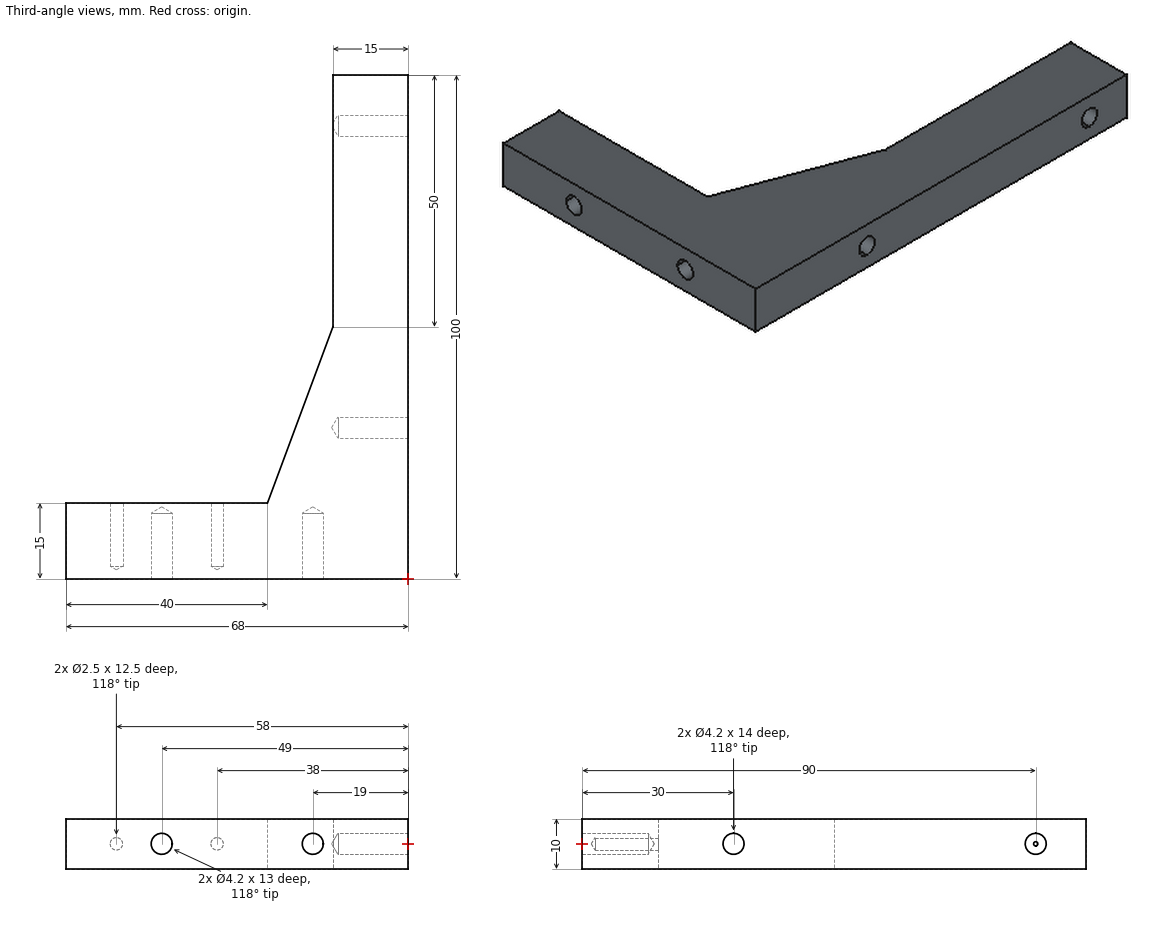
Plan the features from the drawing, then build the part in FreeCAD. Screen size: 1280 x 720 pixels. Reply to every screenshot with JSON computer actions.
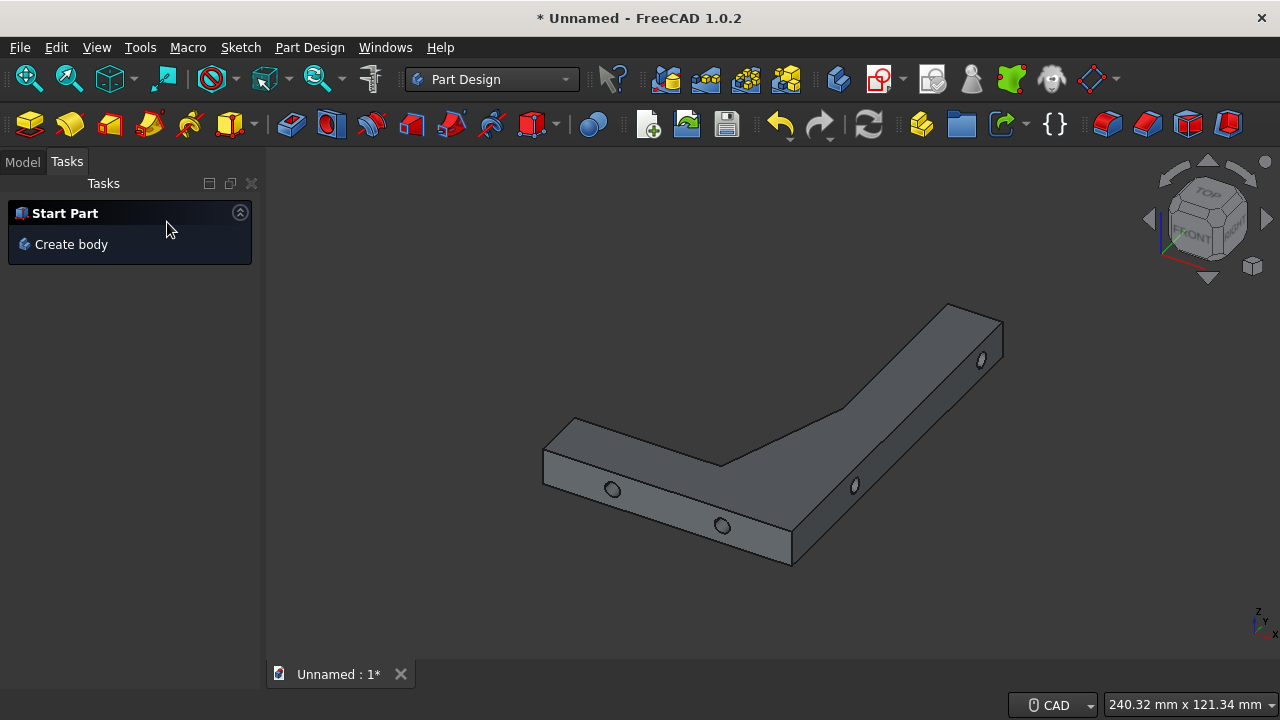
{"action": "key", "text": "4"}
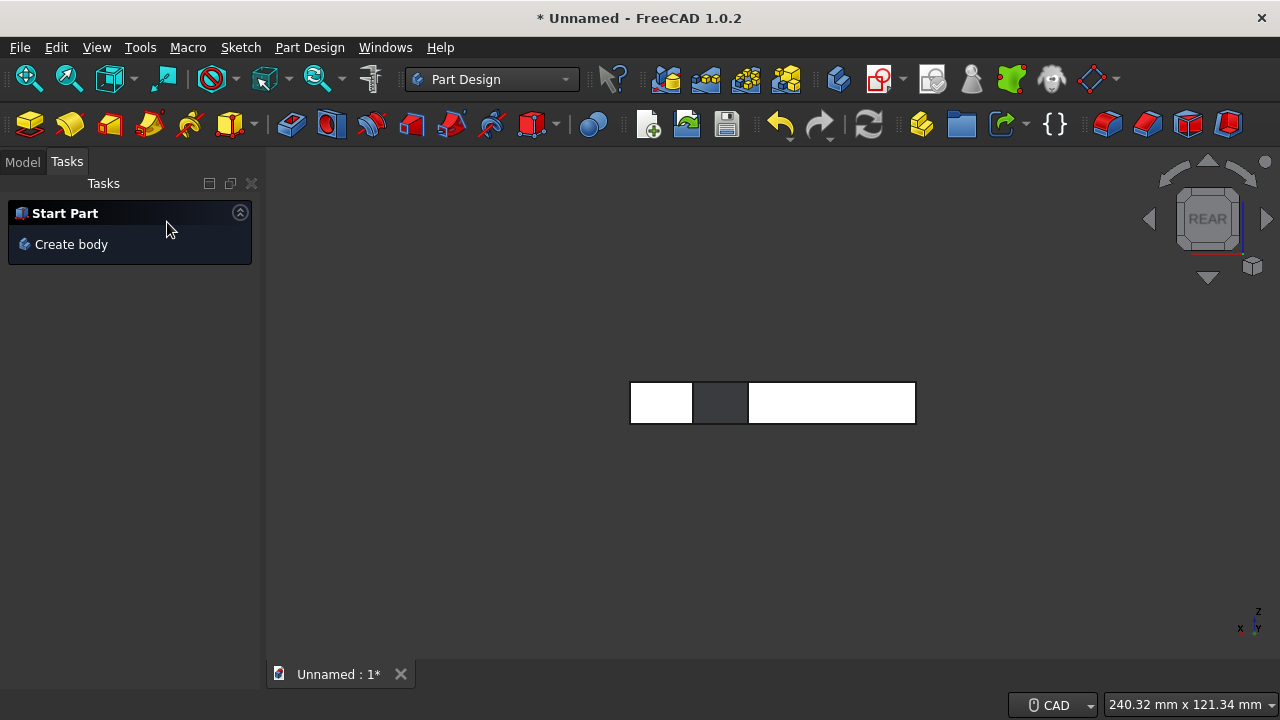
{"action": "key", "text": "v f"}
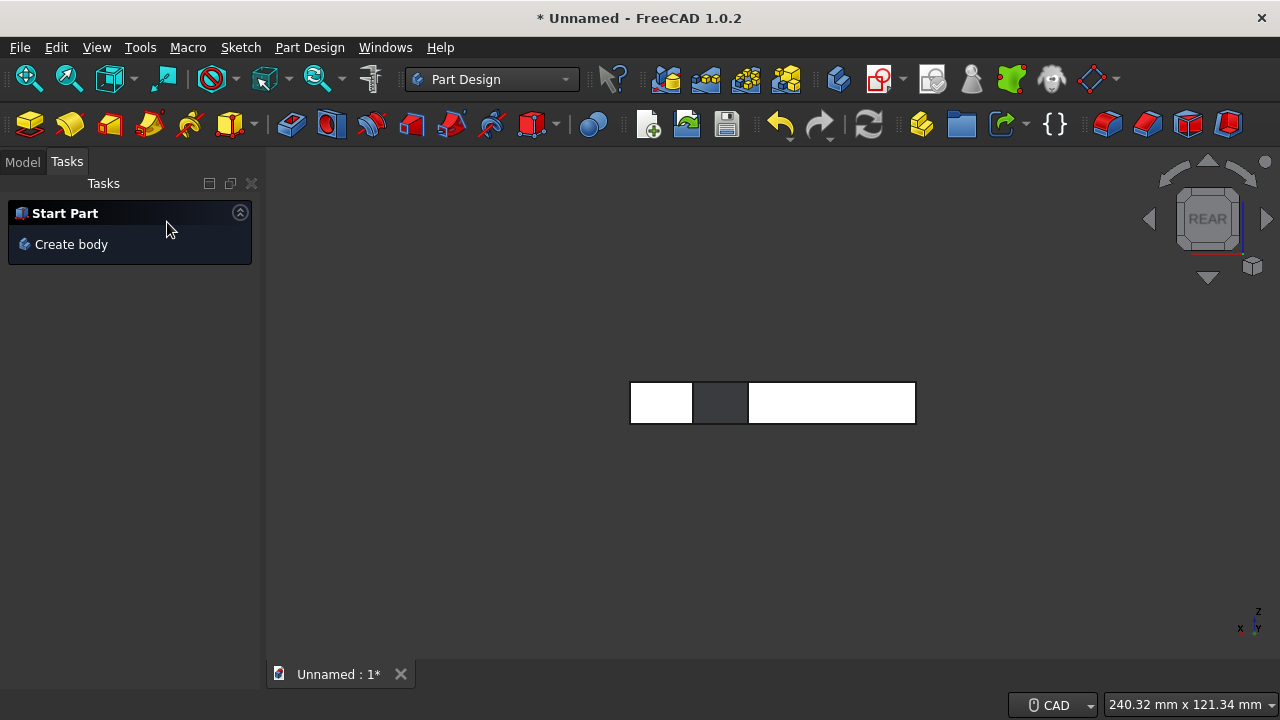
{"action": "left_click", "coordinate": [784, 402]}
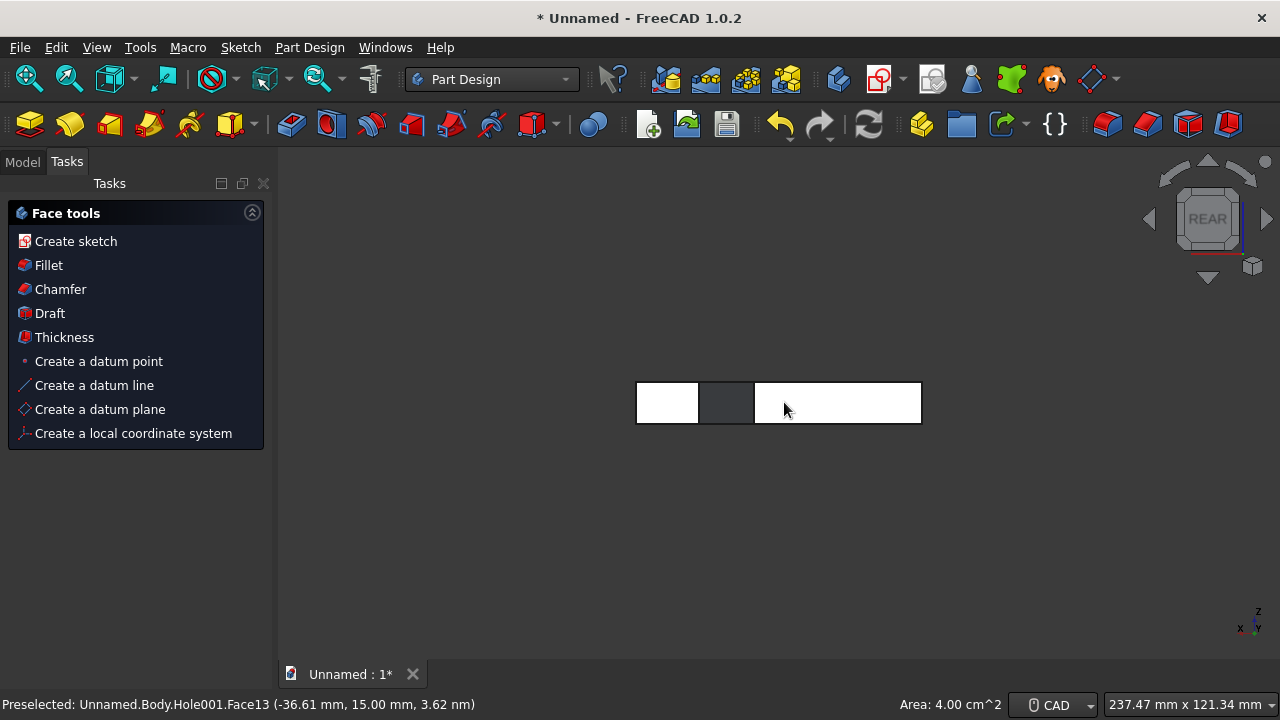
{"action": "left_click", "coordinate": [880, 80]}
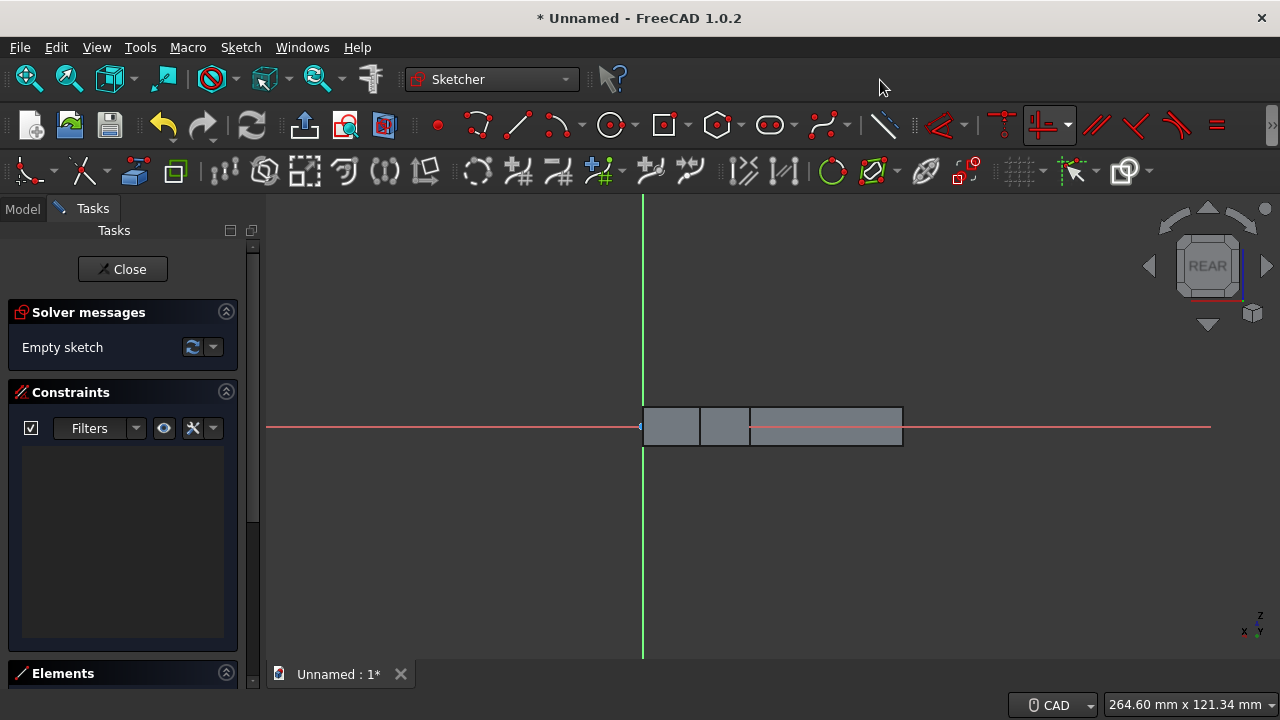
{"action": "scroll", "coordinate": [846, 427], "scroll_direction": "up", "scroll_amount": 10}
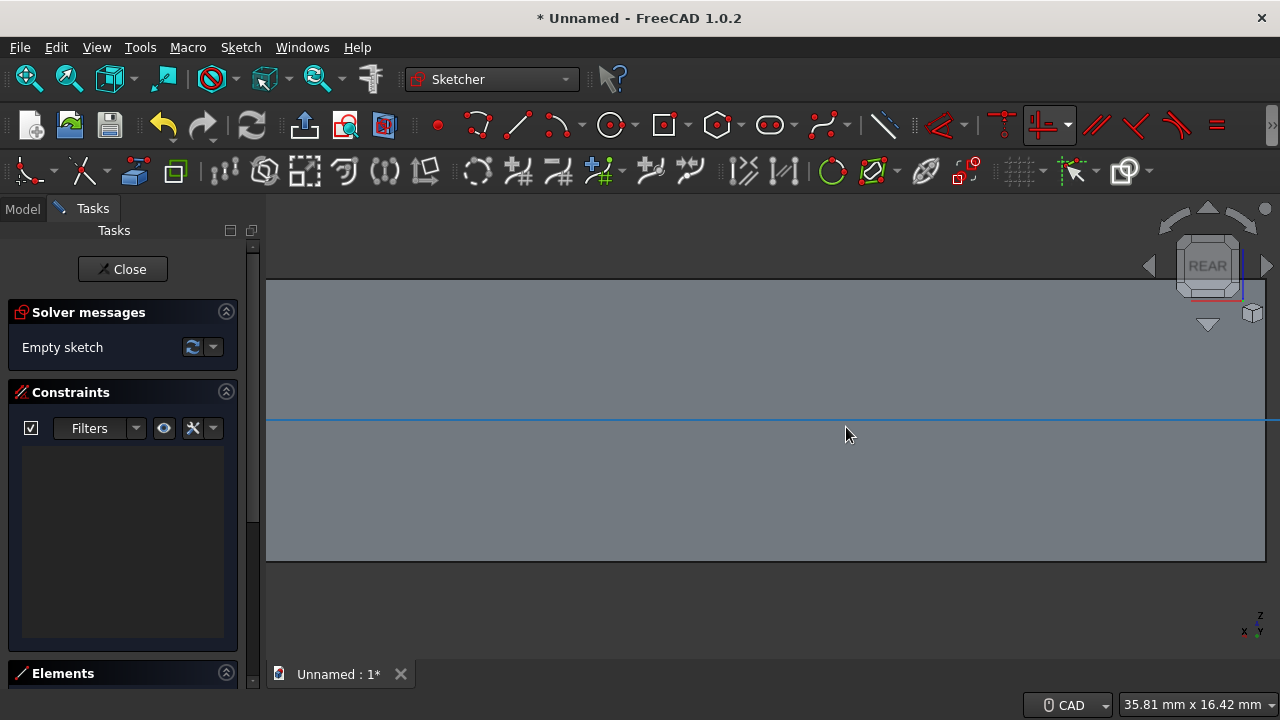
{"action": "key", "text": "g c"}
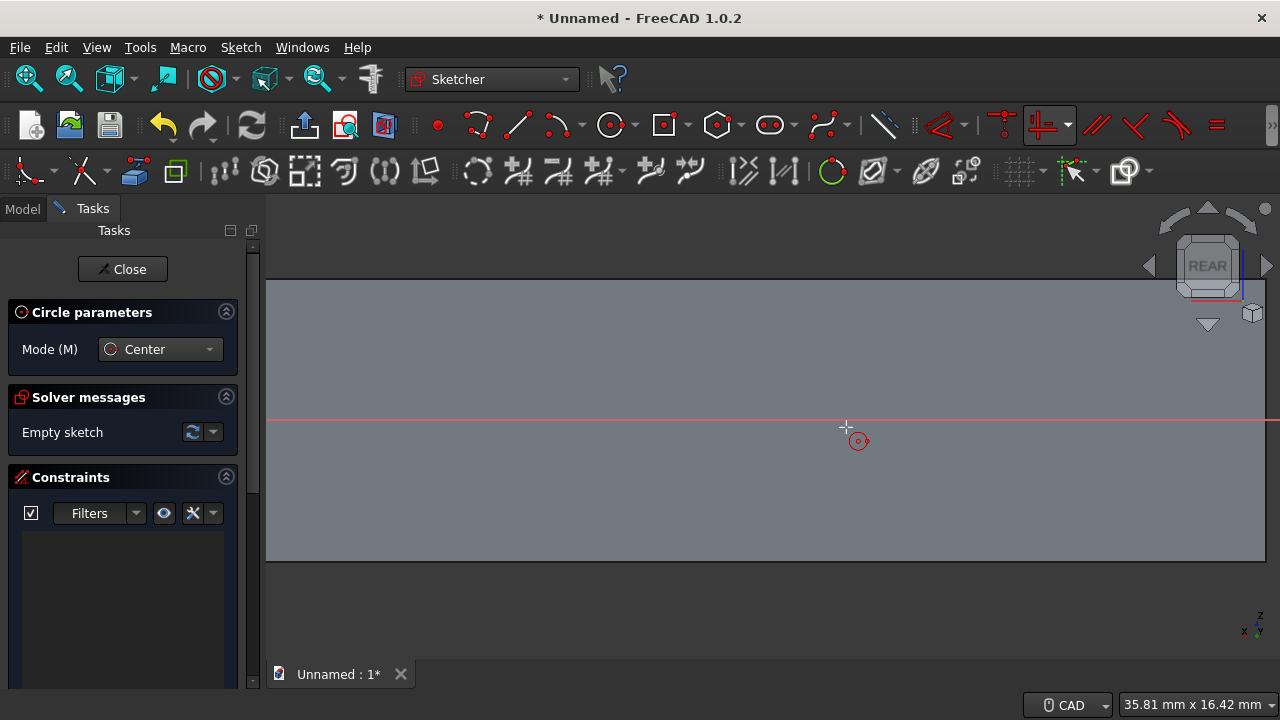
{"action": "left_click", "coordinate": [983, 420]}
{"action": "mouse_move", "coordinate": [1008, 395]}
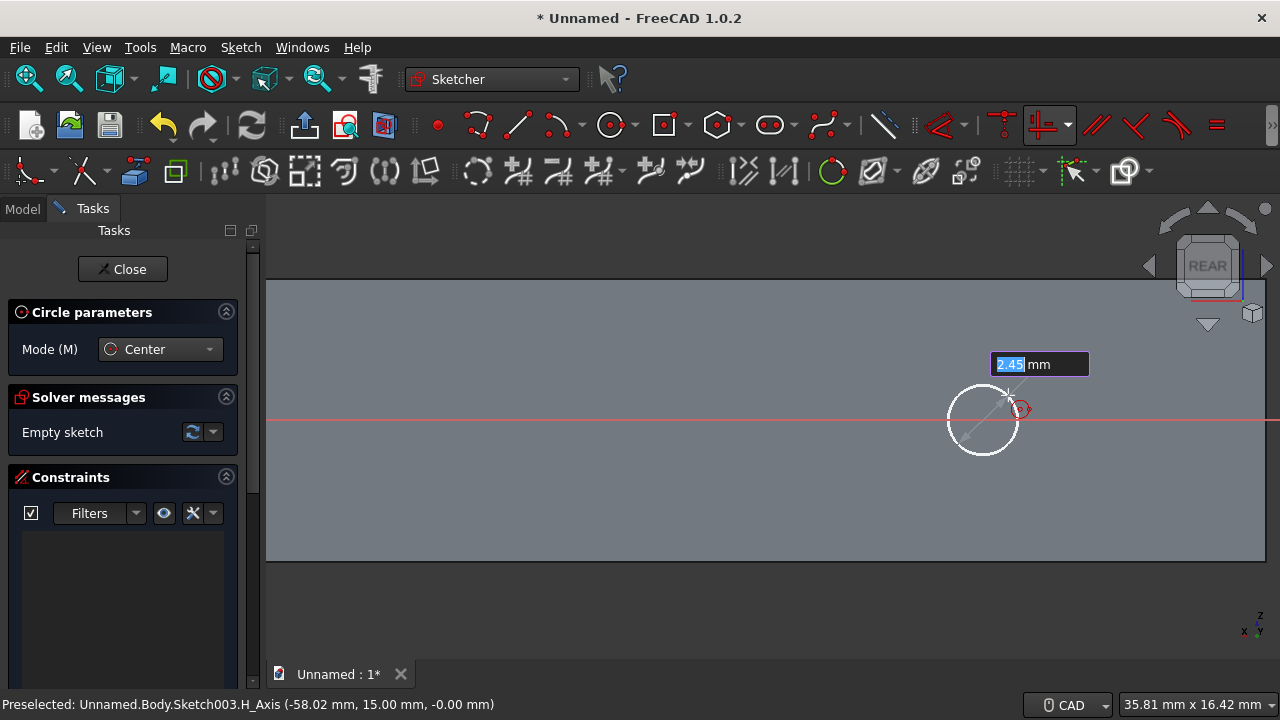
{"action": "type", "text": "2.5"}
{"action": "key", "text": "Return"}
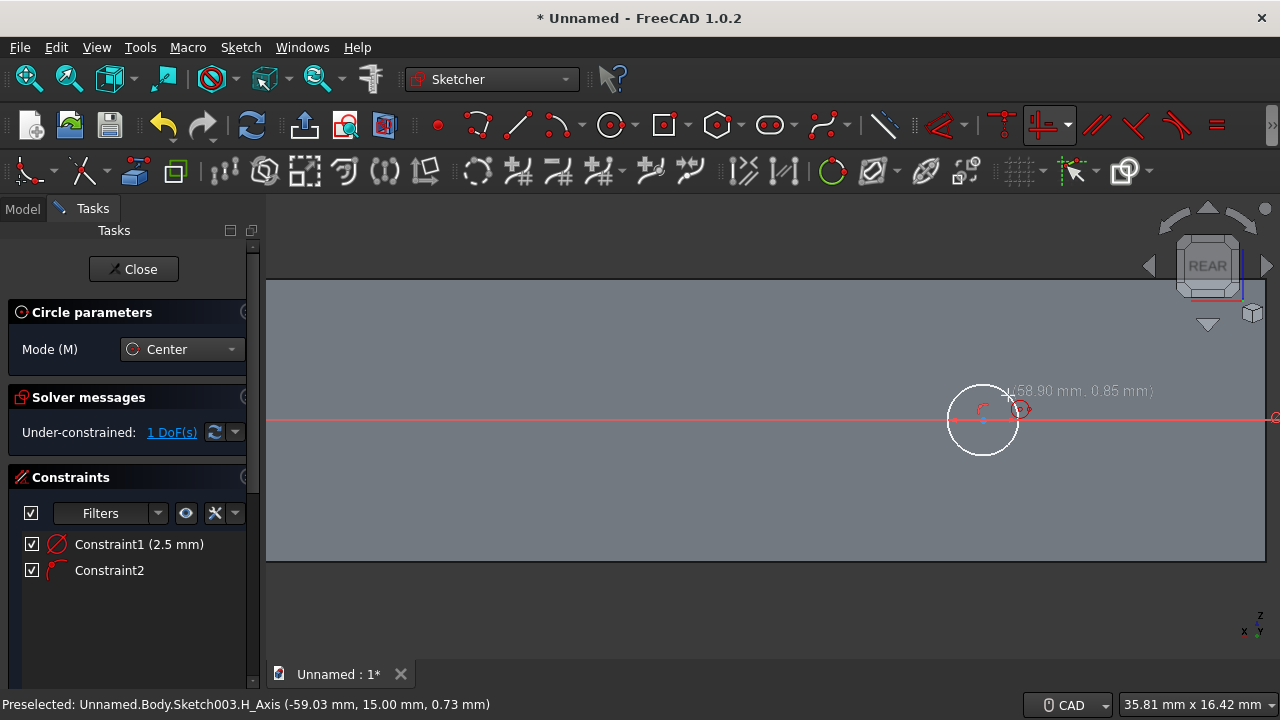
{"action": "left_click", "coordinate": [416, 420]}
{"action": "mouse_move", "coordinate": [441, 395]}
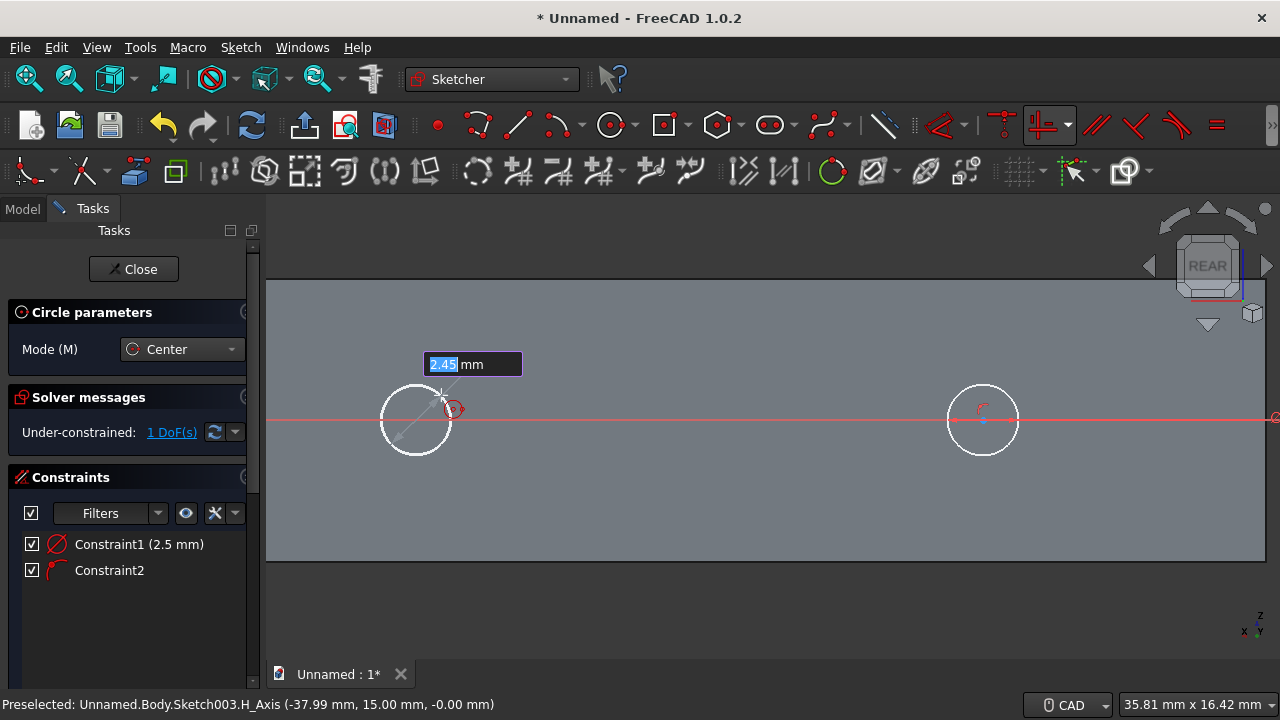
{"action": "type", "text": "2.5"}
{"action": "key", "text": "Return"}
{"action": "key", "text": "Escape"}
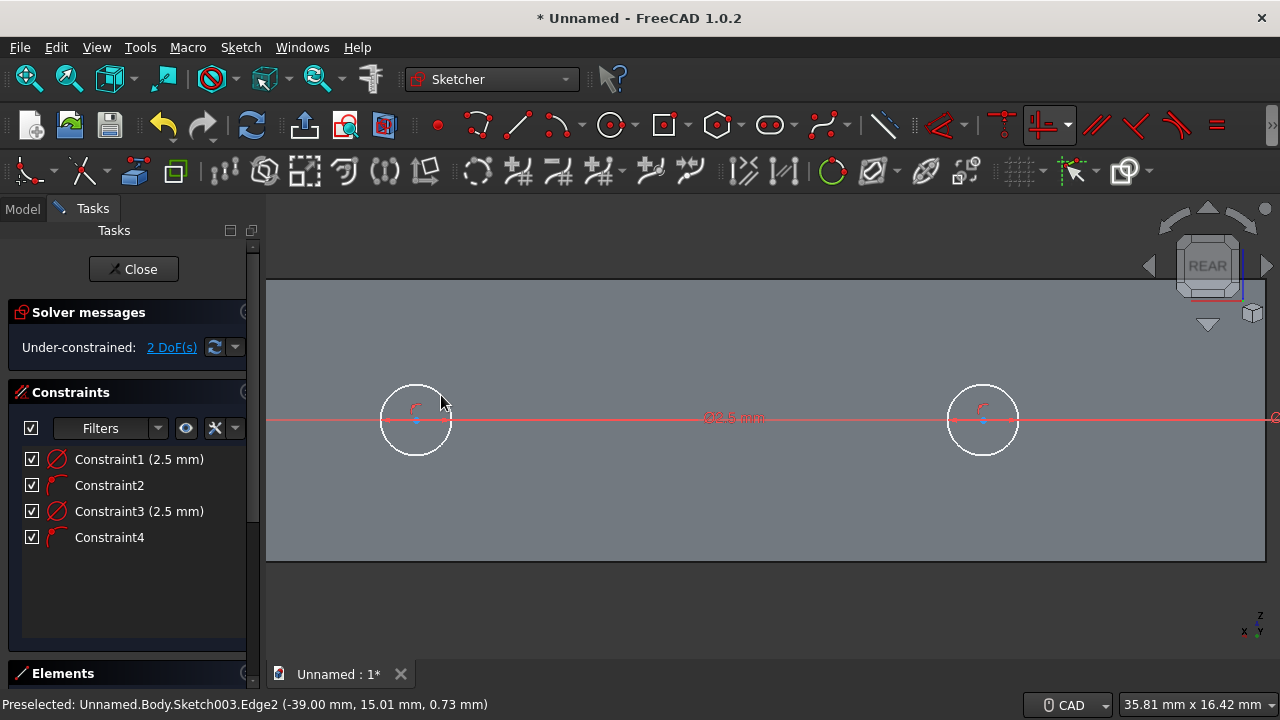
{"action": "key", "text": "d"}